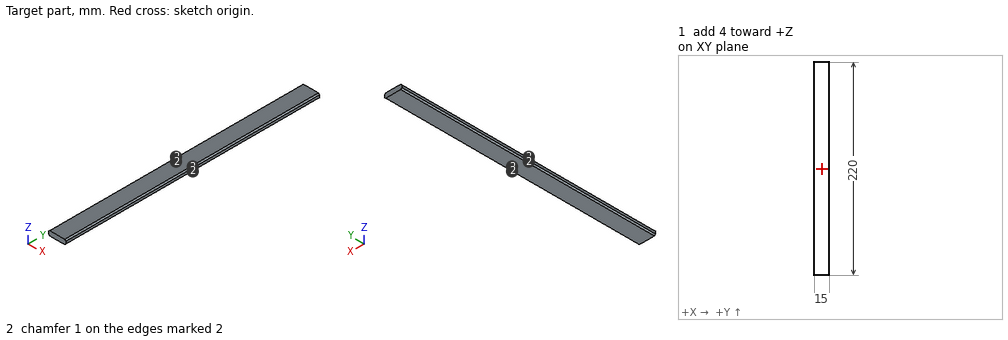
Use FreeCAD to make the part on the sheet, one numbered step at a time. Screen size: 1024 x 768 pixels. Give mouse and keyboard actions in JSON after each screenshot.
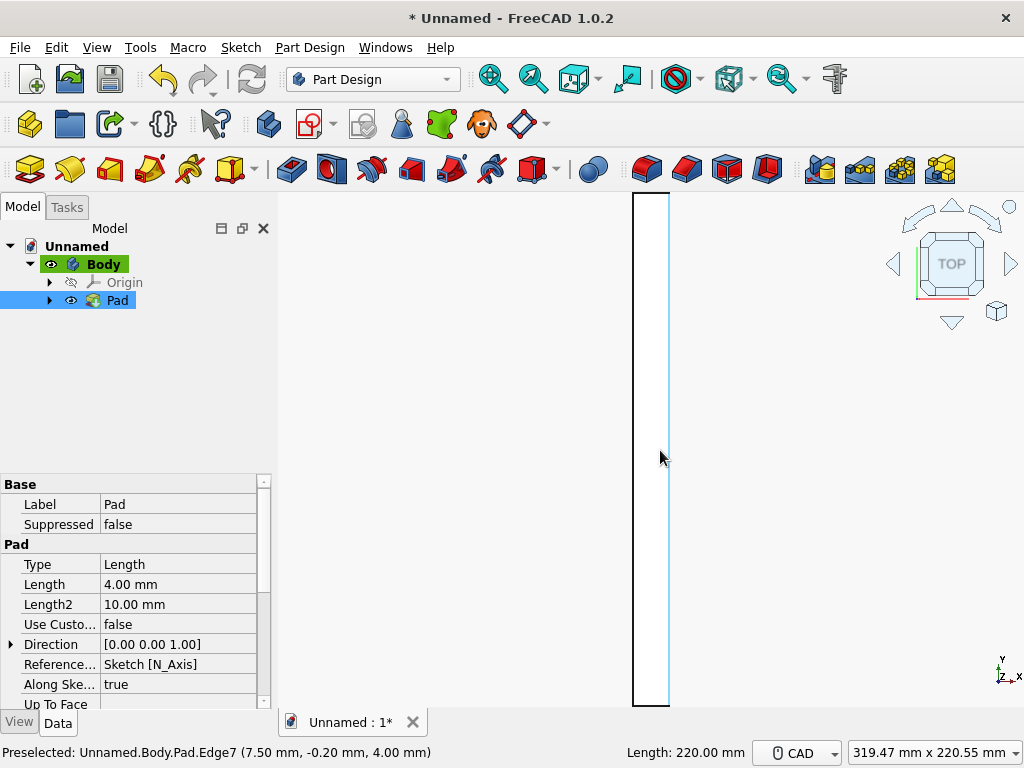
{"action": "left_click", "coordinate": [633, 448], "text": "ctrl"}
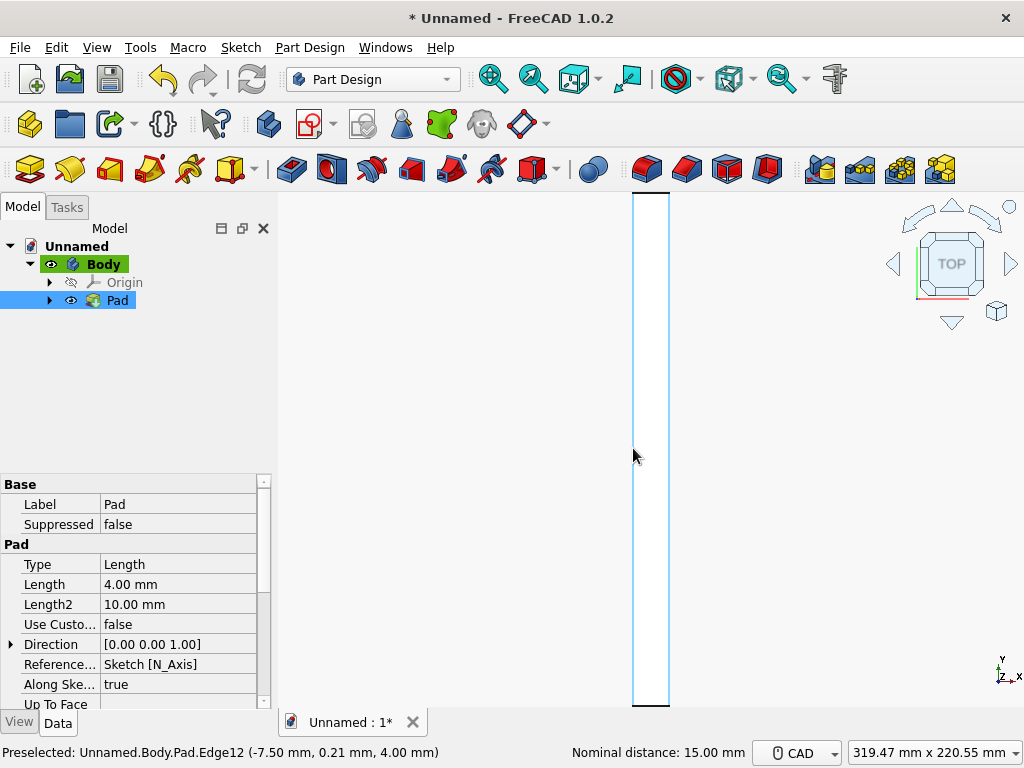
{"action": "key", "text": "1"}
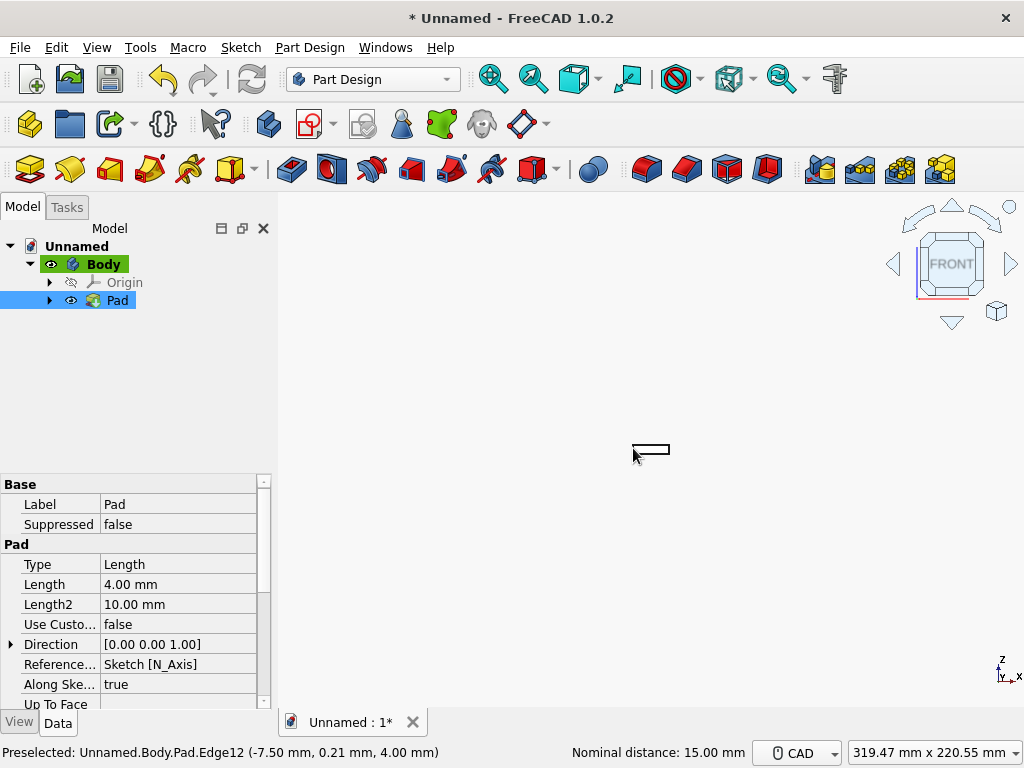
{"action": "key", "text": "v f"}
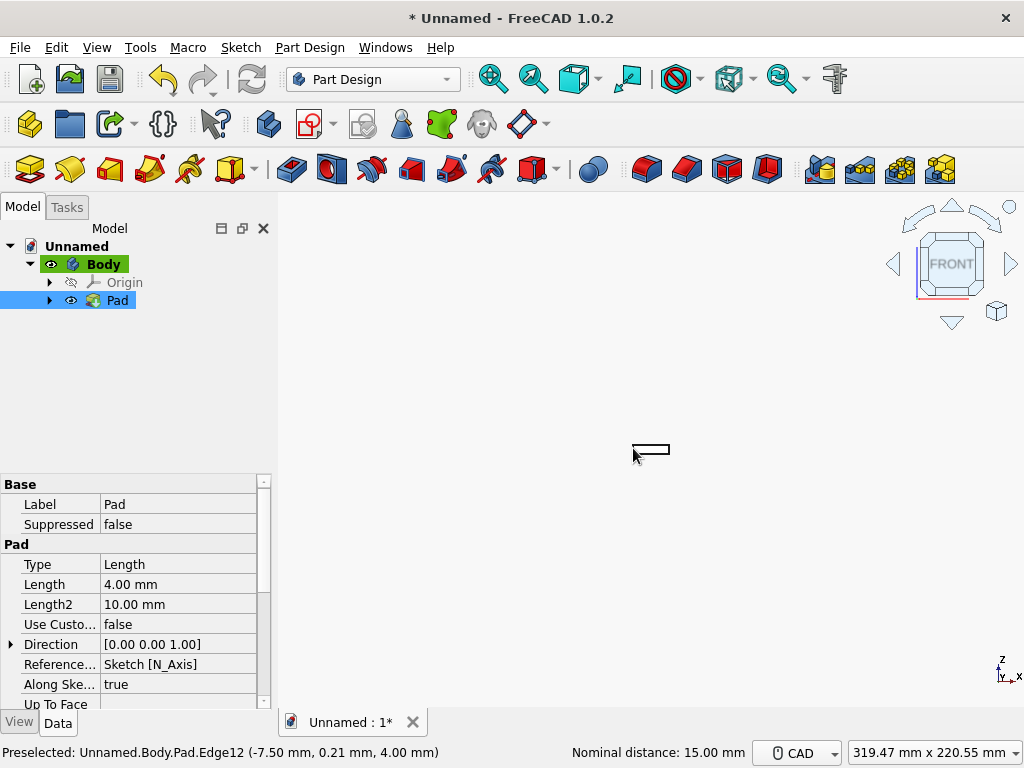
{"action": "key", "text": "3"}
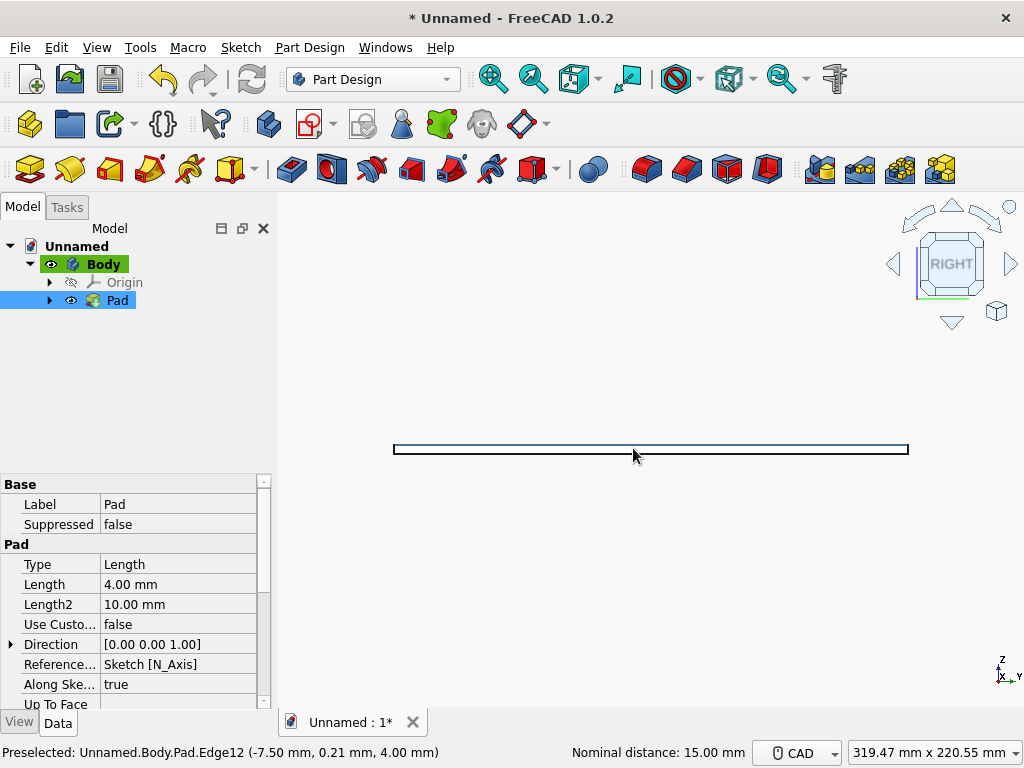
{"action": "left_click", "coordinate": [651, 453], "text": "ctrl"}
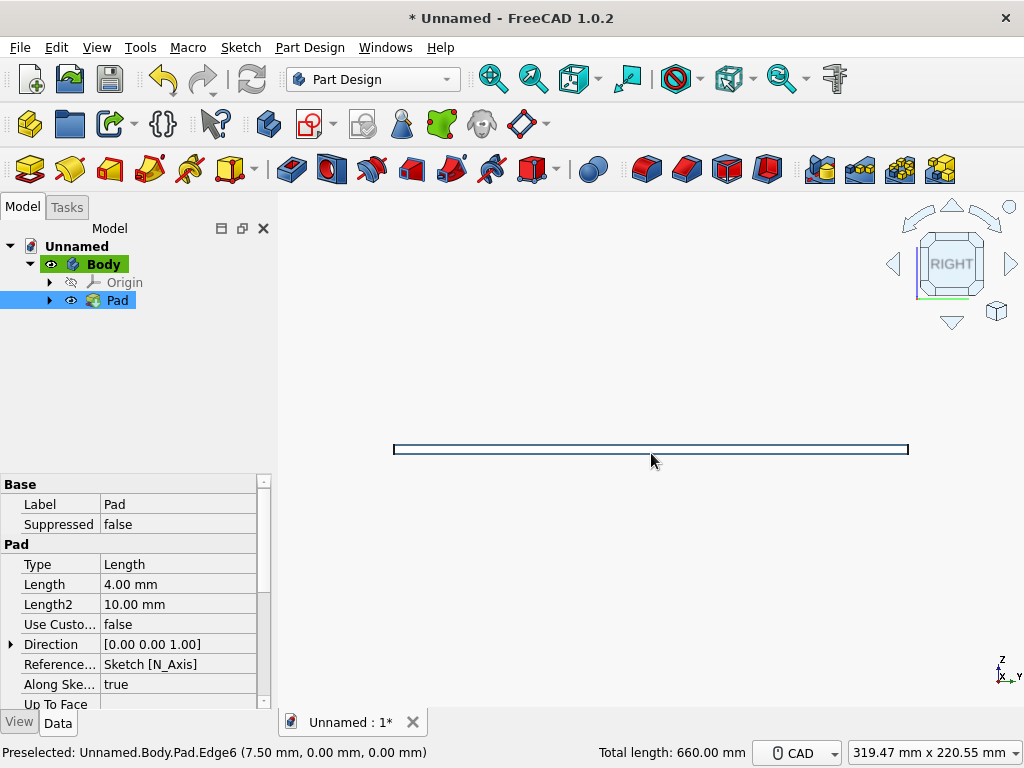
{"action": "key", "text": "5"}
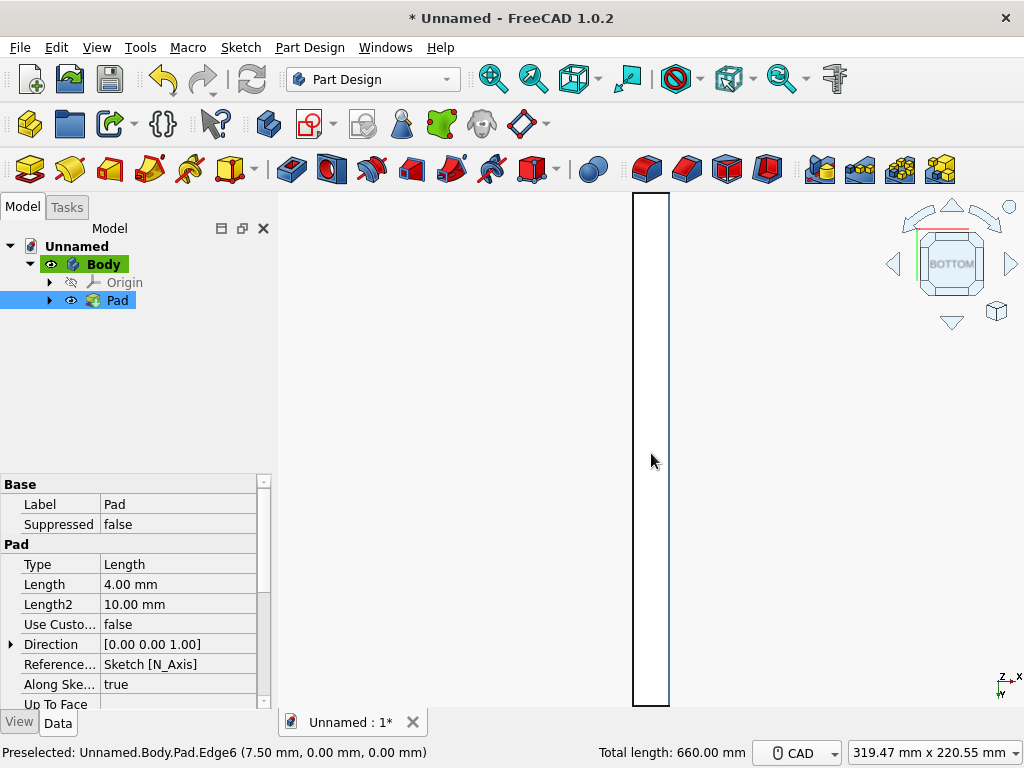
{"action": "left_click", "coordinate": [633, 448], "text": "ctrl"}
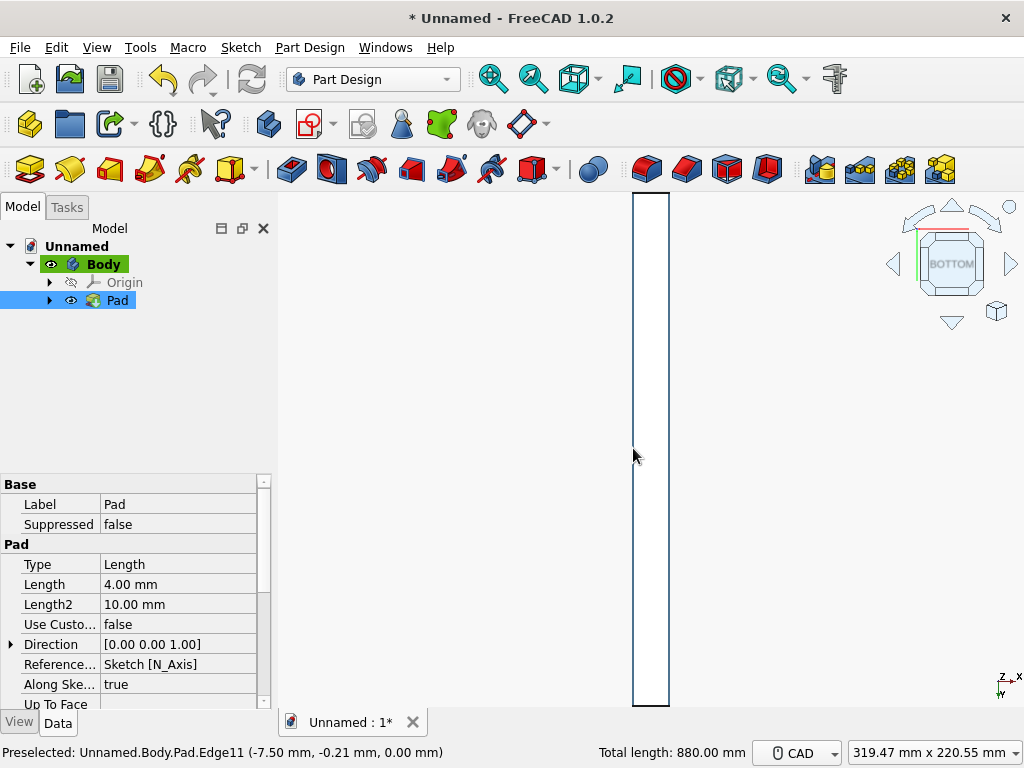
{"action": "left_click", "coordinate": [688, 170]}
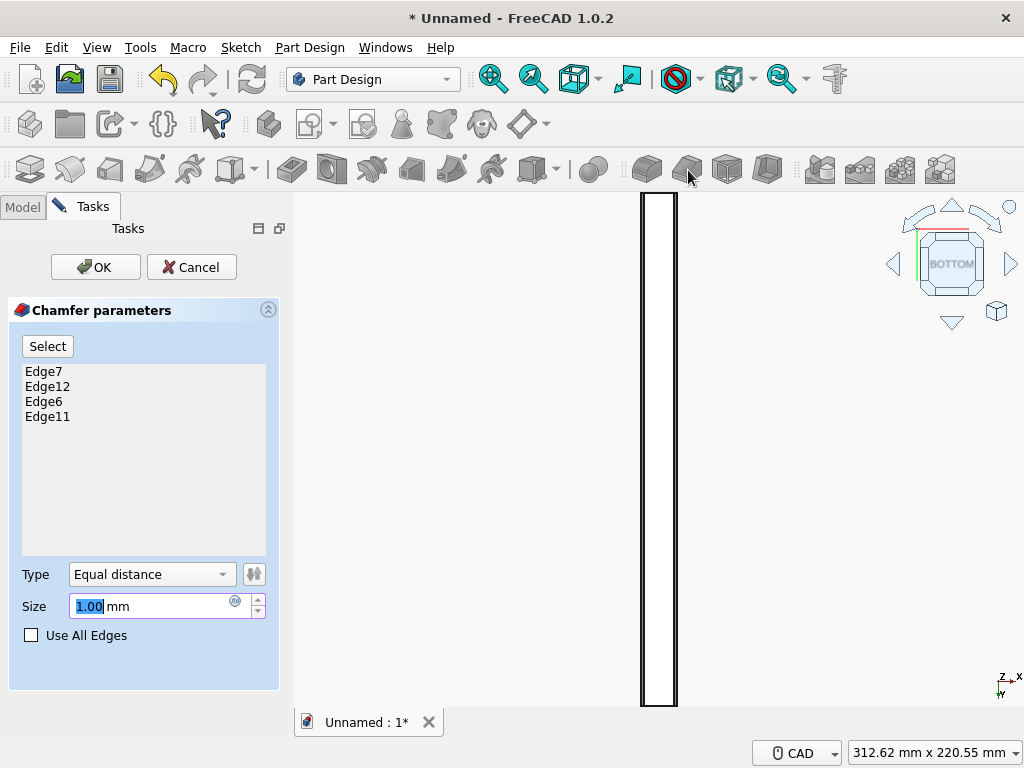
{"action": "type", "text": "1"}
{"action": "key", "text": "Tab"}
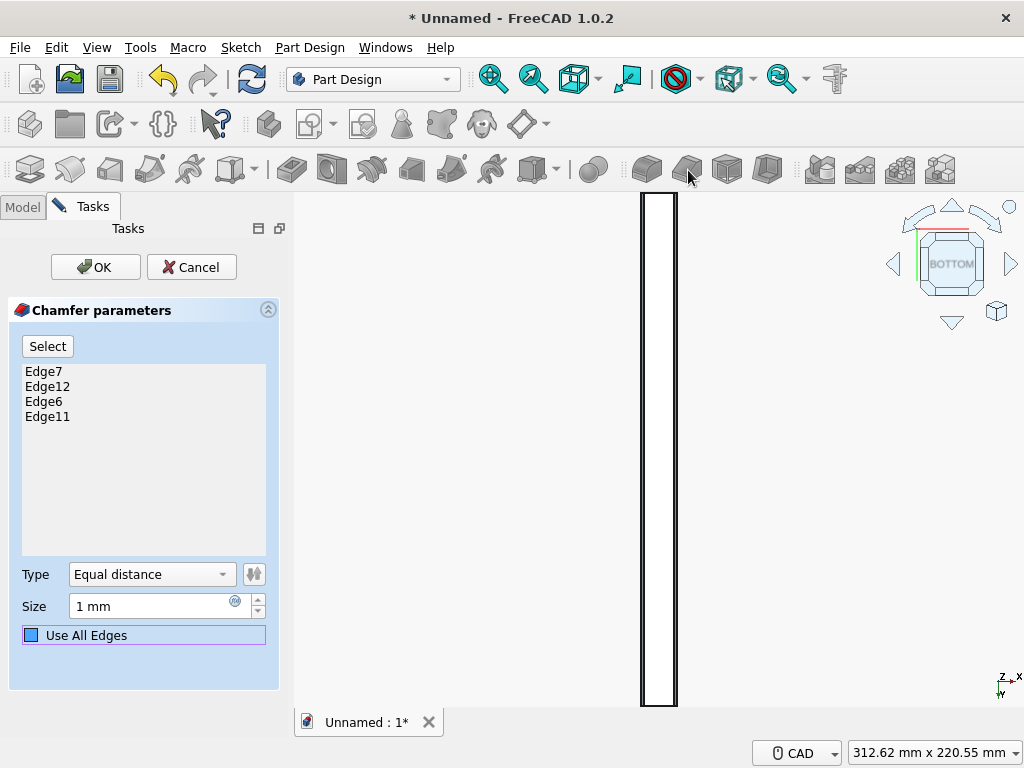
{"action": "left_click", "coordinate": [96, 267]}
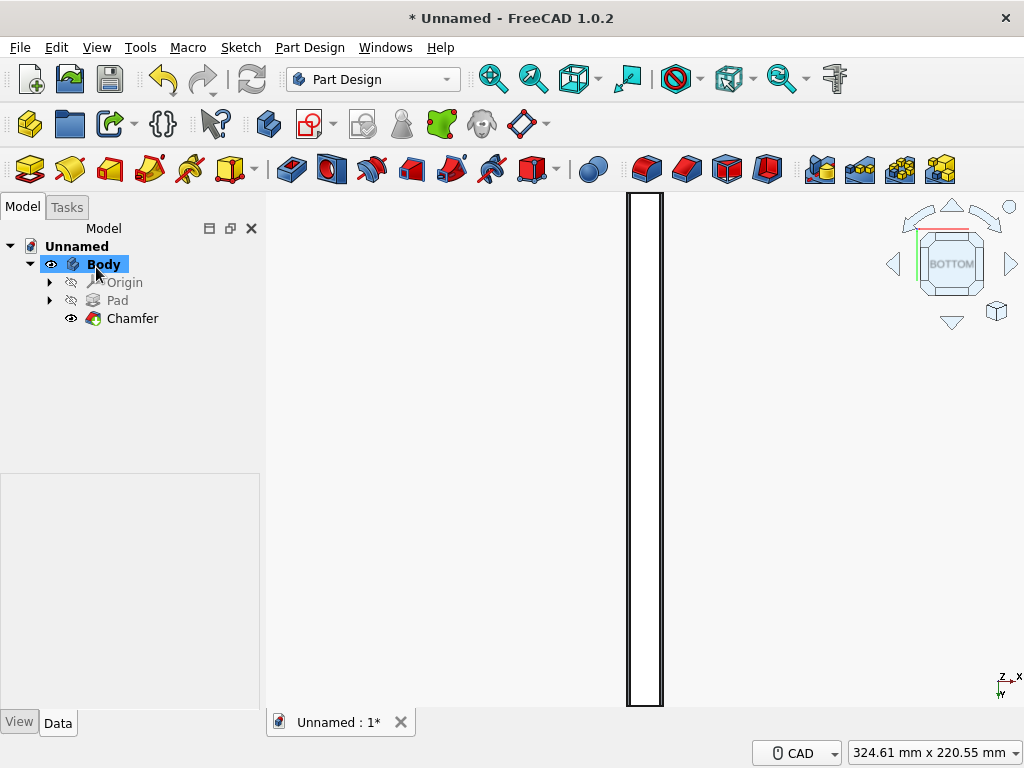
{"action": "key", "text": "0"}